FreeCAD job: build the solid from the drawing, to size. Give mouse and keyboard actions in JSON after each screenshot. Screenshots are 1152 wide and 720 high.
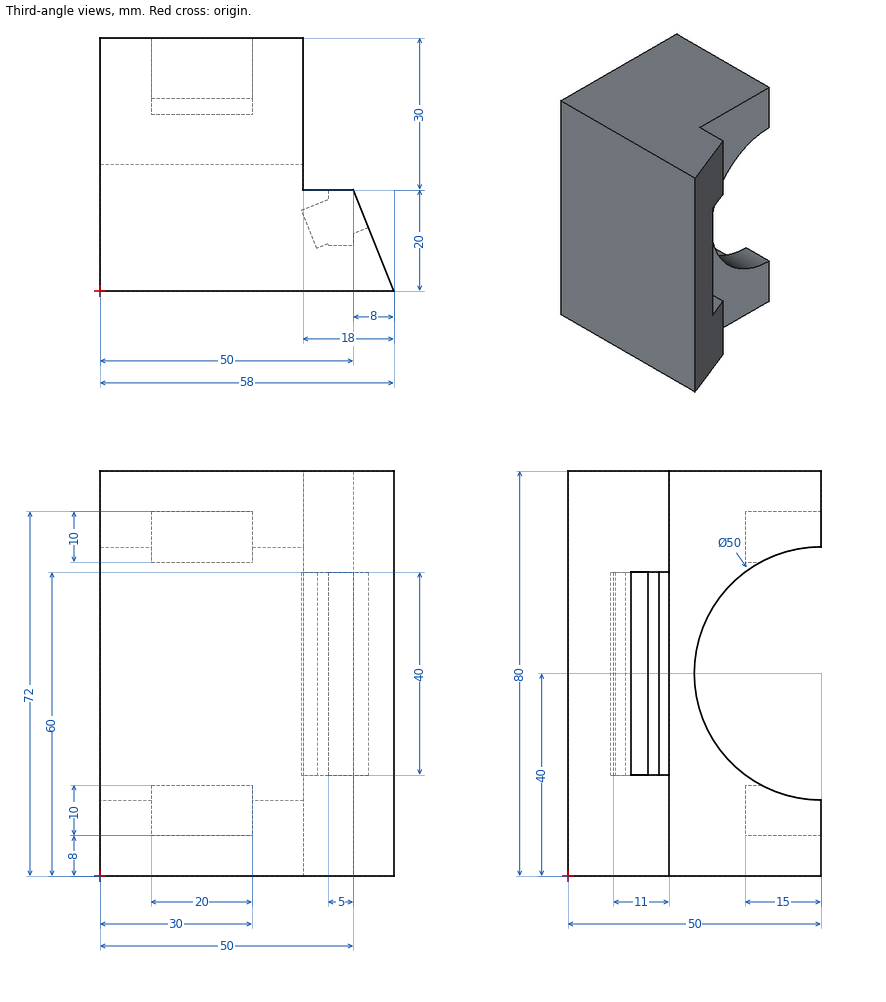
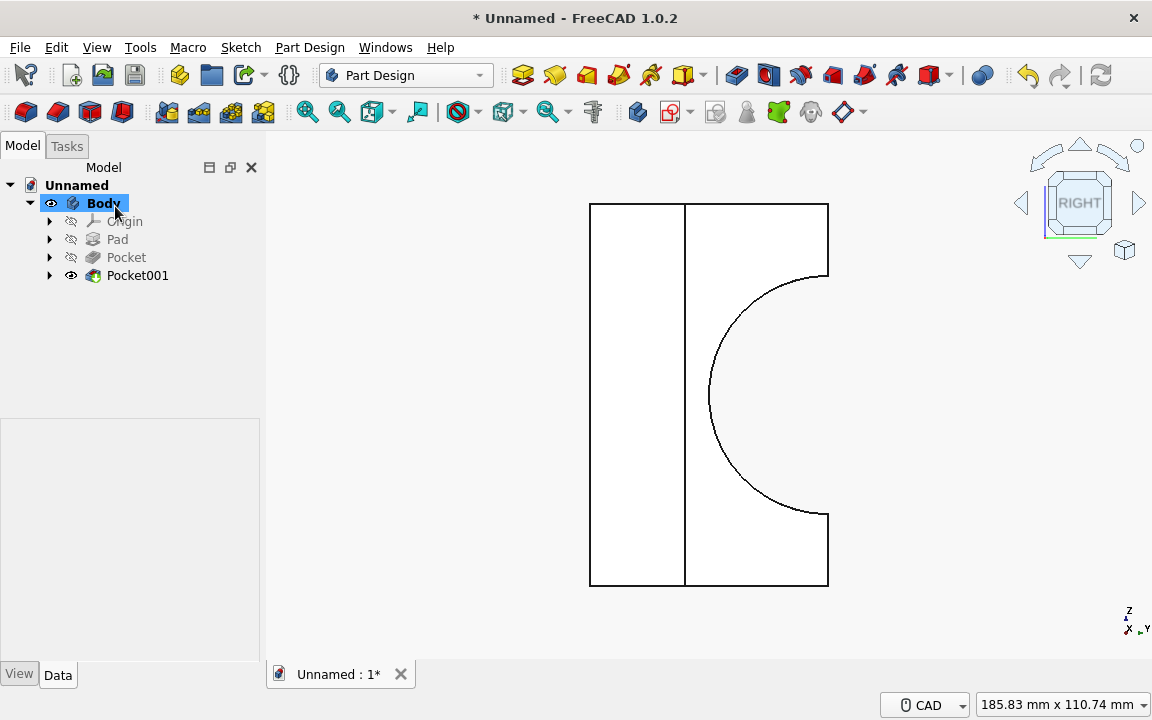
{"action": "key", "text": "0"}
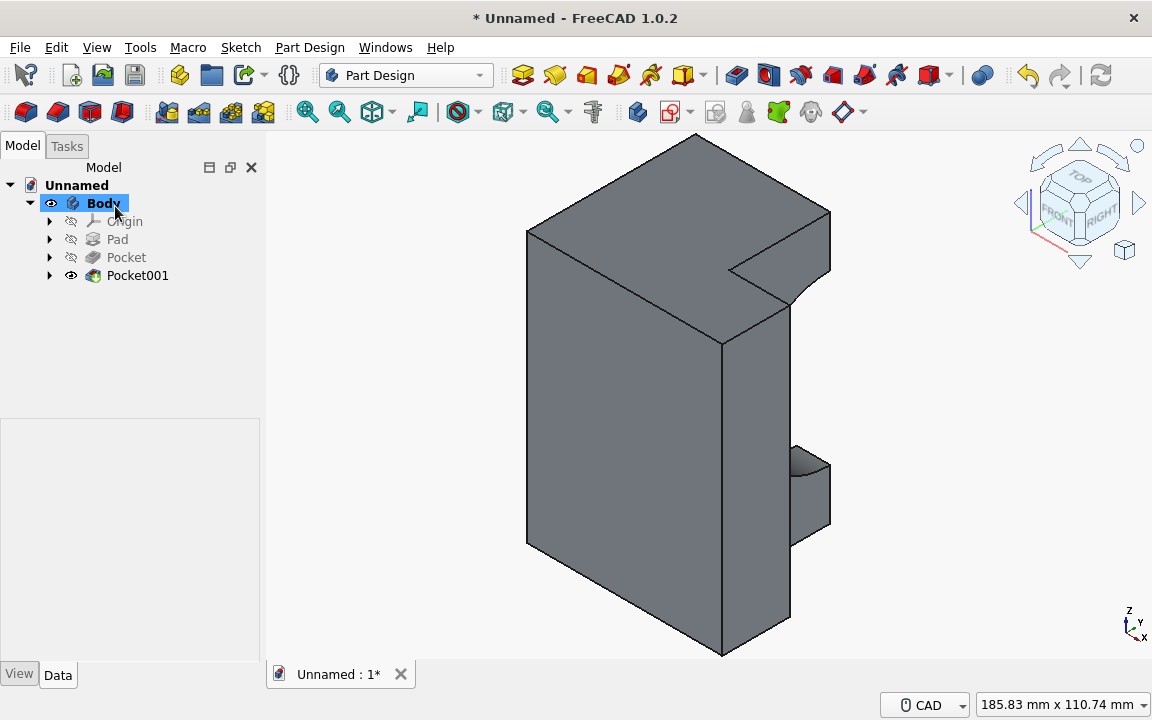
{"action": "left_click", "coordinate": [681, 222]}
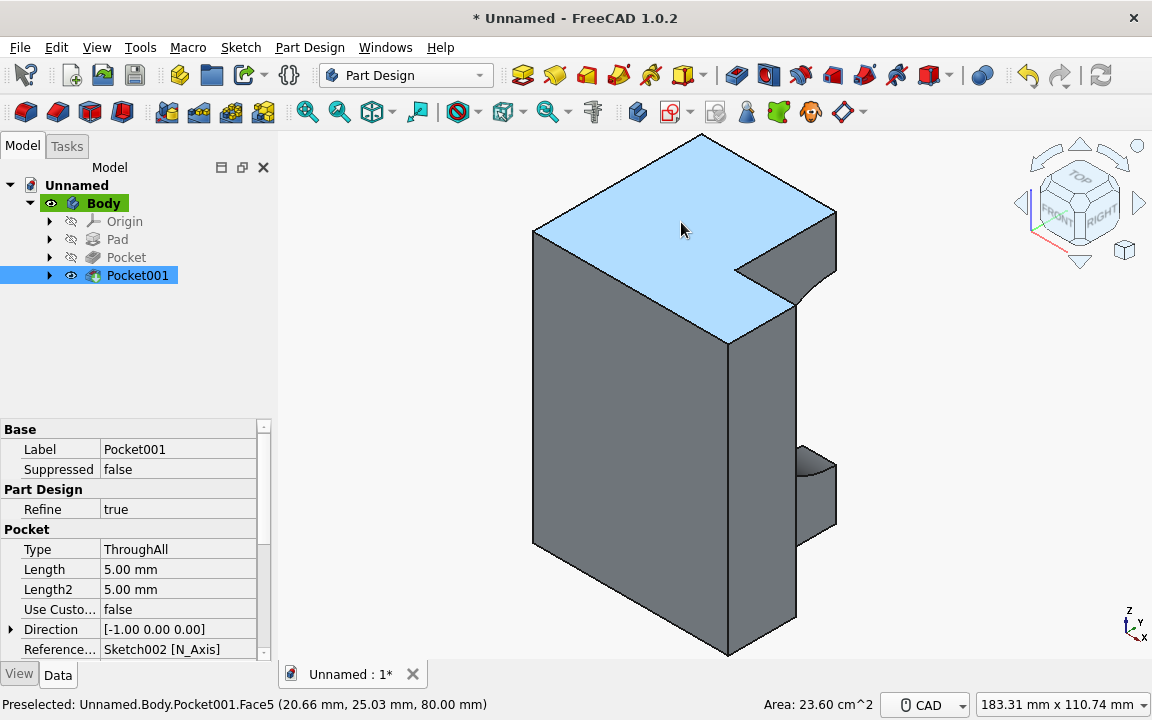
{"action": "left_click", "coordinate": [670, 112]}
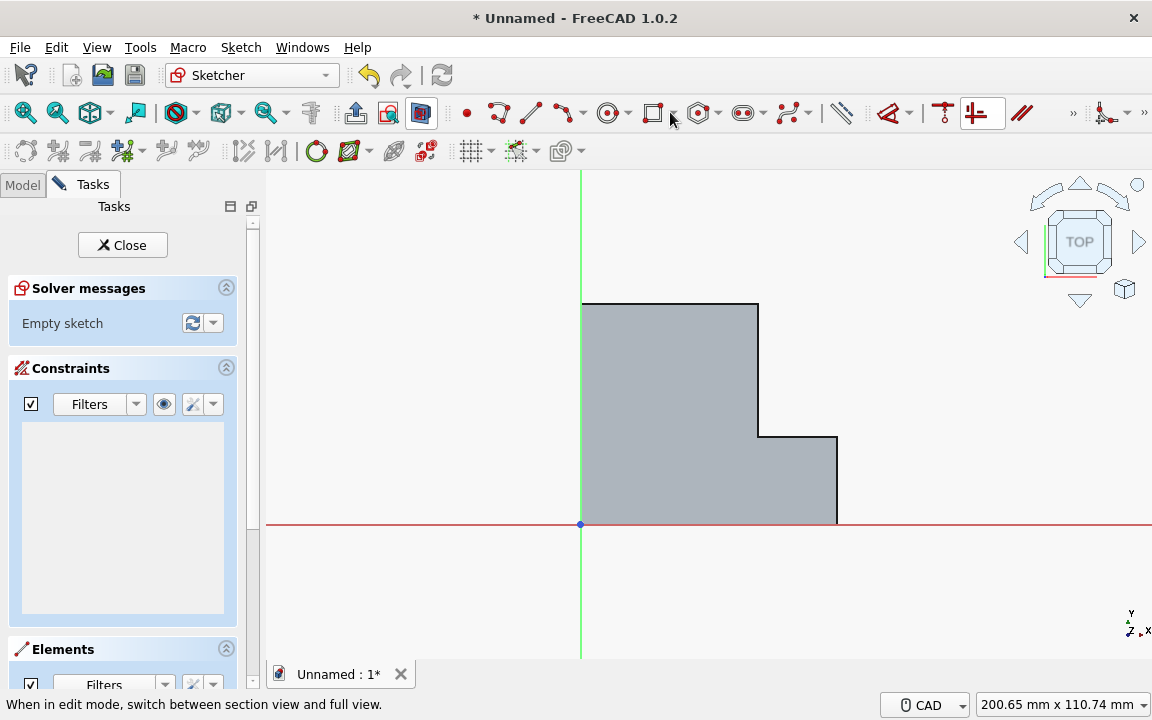
{"action": "scroll", "coordinate": [896, 509], "scroll_direction": "up", "scroll_amount": 6}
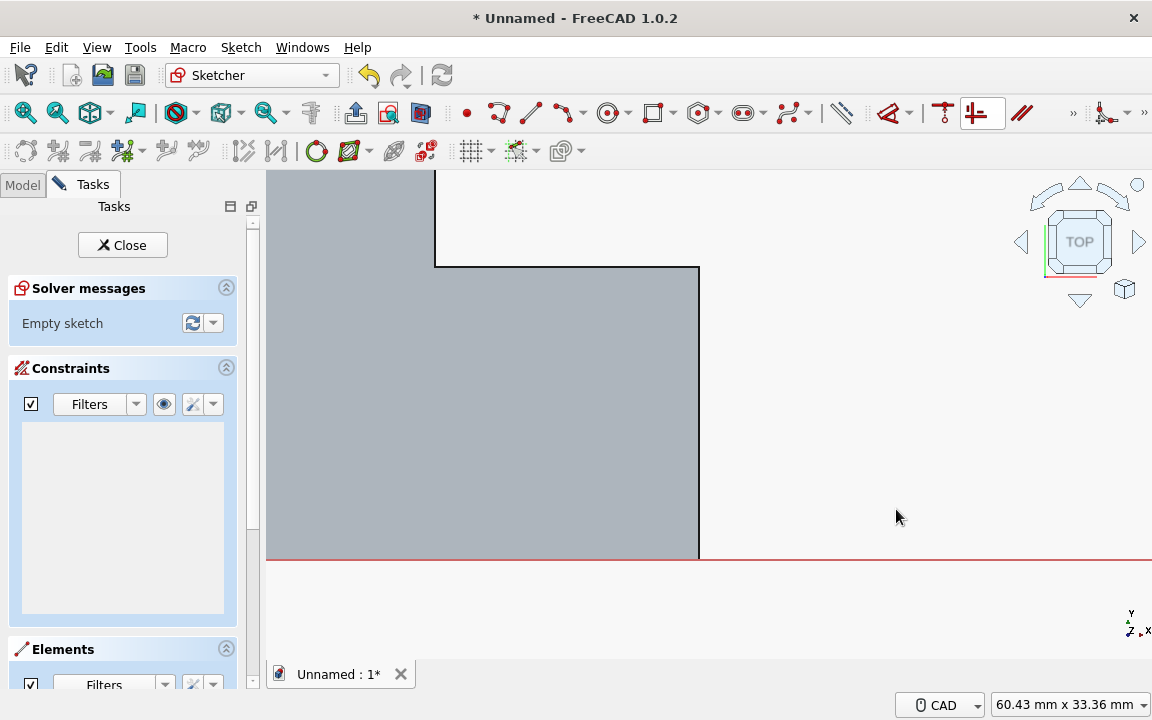
{"action": "left_click", "coordinate": [500, 114]}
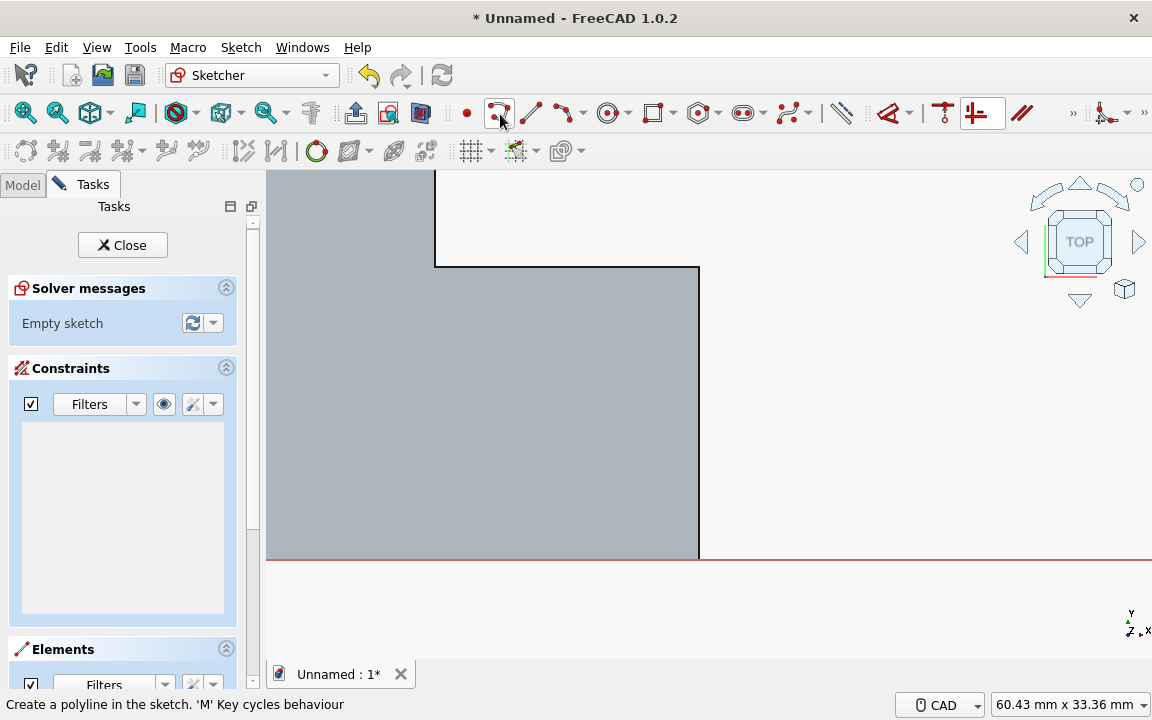
{"action": "left_click", "coordinate": [581, 267]}
{"action": "left_click", "coordinate": [699, 560]}
{"action": "left_click", "coordinate": [699, 267]}
{"action": "left_click", "coordinate": [581, 268]}
{"action": "key", "text": "Escape"}
{"action": "key", "text": "Escape"}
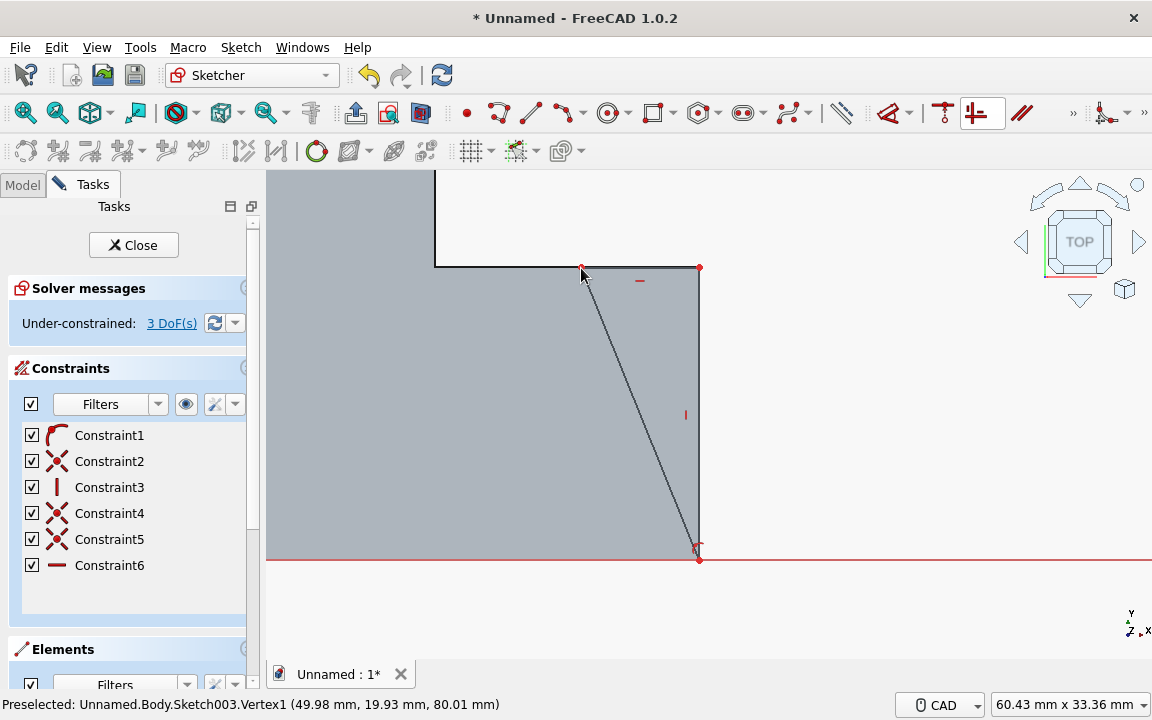
{"action": "left_click", "coordinate": [888, 114]}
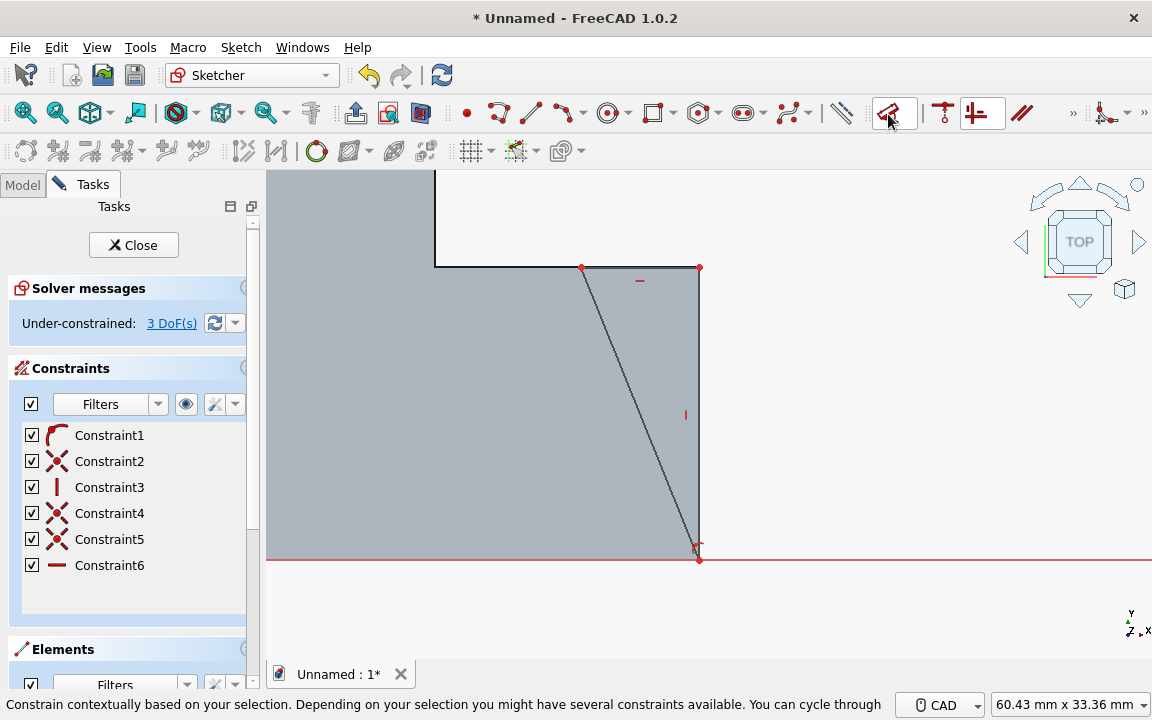
{"action": "left_click", "coordinate": [664, 268]}
{"action": "left_click", "coordinate": [640, 234]}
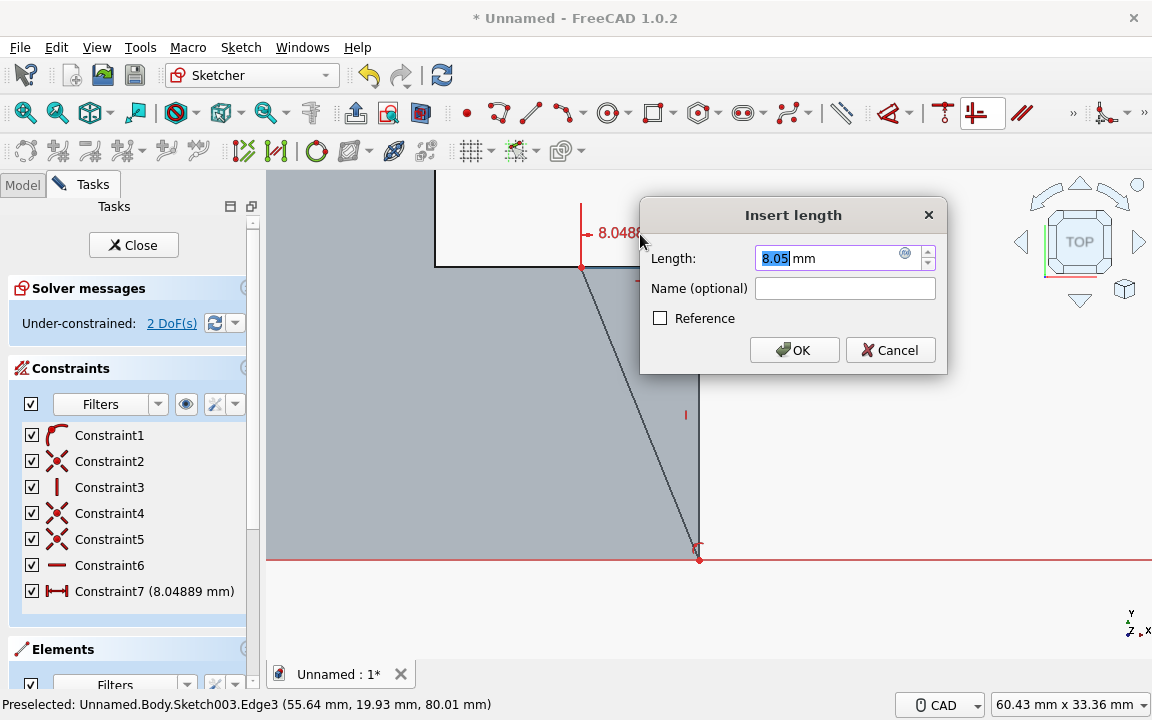
{"action": "type", "text": "8"}
{"action": "key", "text": "Return"}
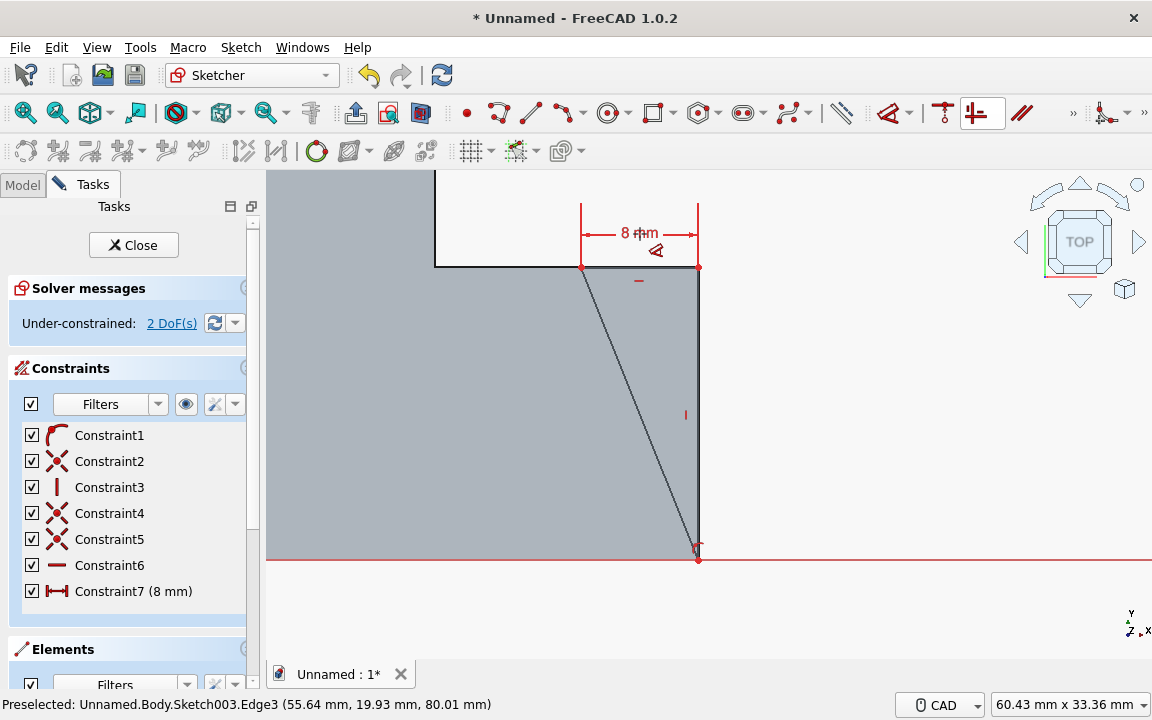
{"action": "left_click", "coordinate": [698, 473]}
{"action": "left_click", "coordinate": [732, 414]}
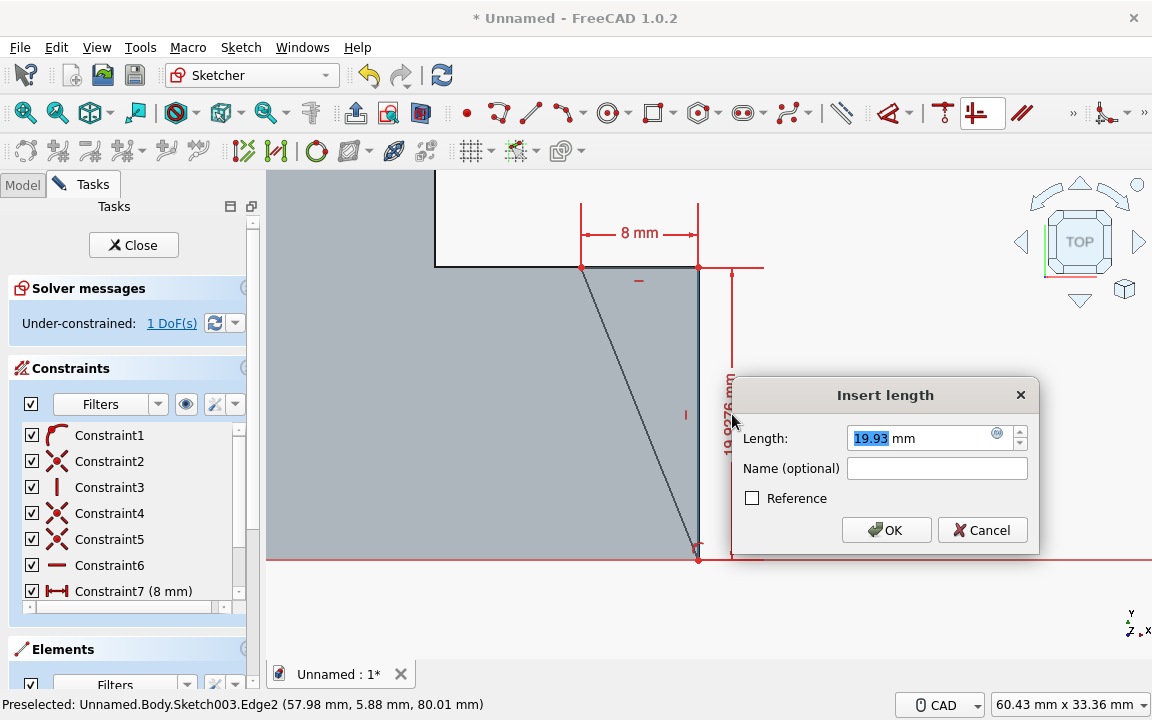
{"action": "type", "text": "20"}
{"action": "key", "text": "Return"}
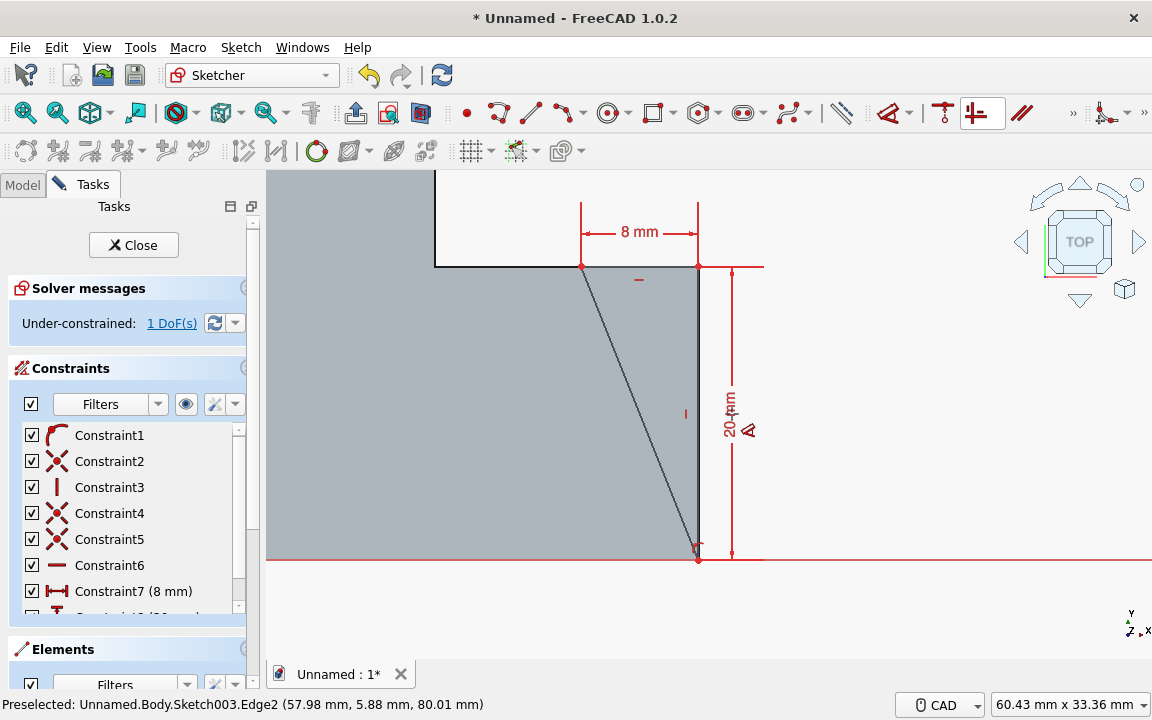
{"action": "left_click", "coordinate": [581, 267]}
{"action": "left_click", "coordinate": [437, 594]}